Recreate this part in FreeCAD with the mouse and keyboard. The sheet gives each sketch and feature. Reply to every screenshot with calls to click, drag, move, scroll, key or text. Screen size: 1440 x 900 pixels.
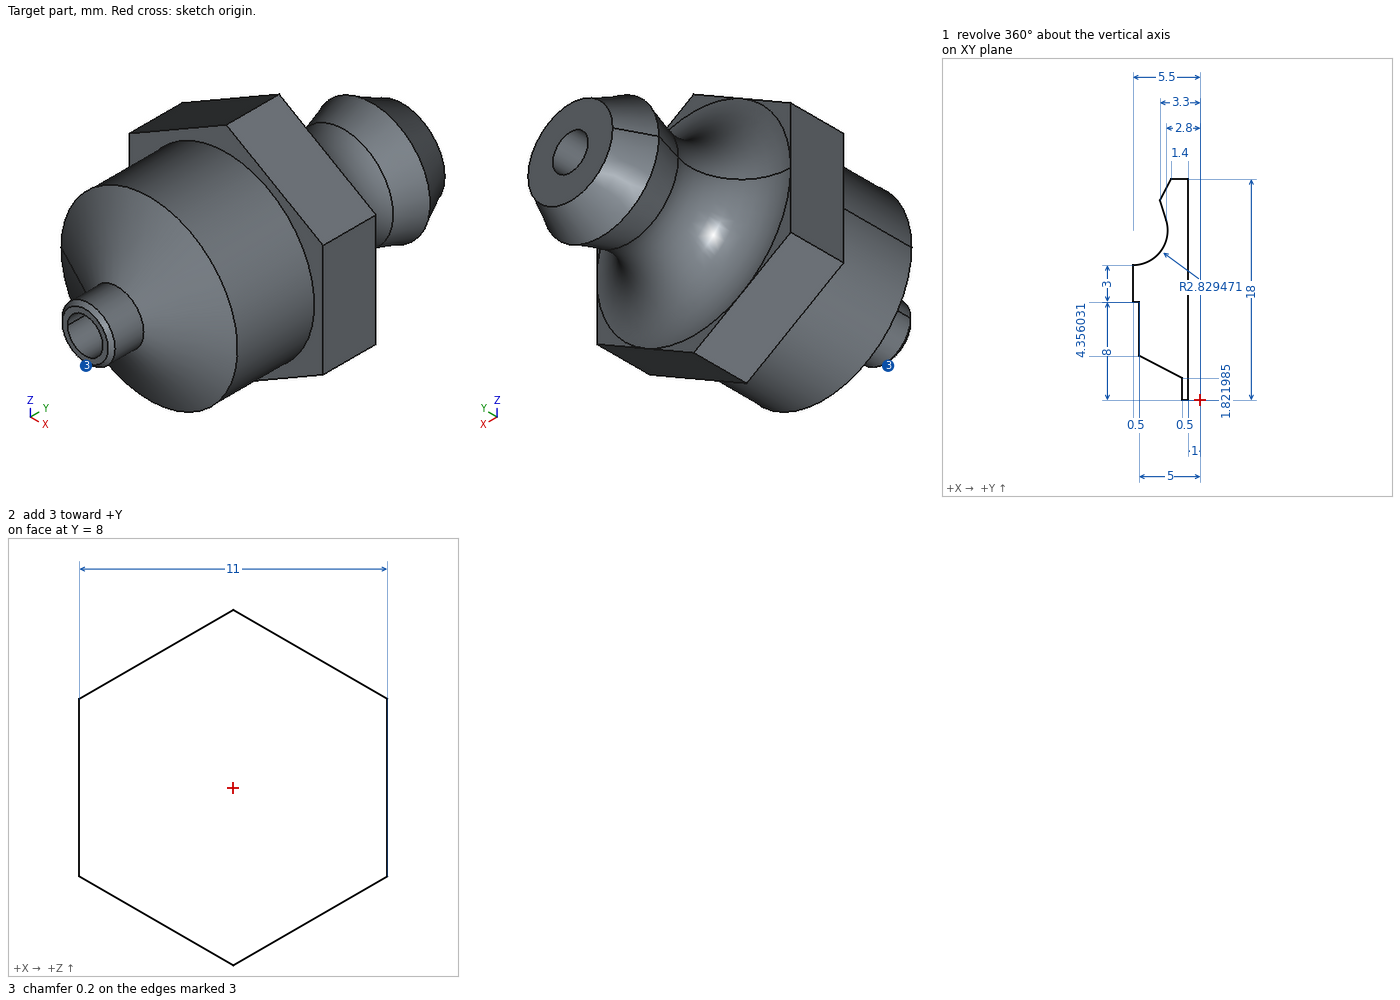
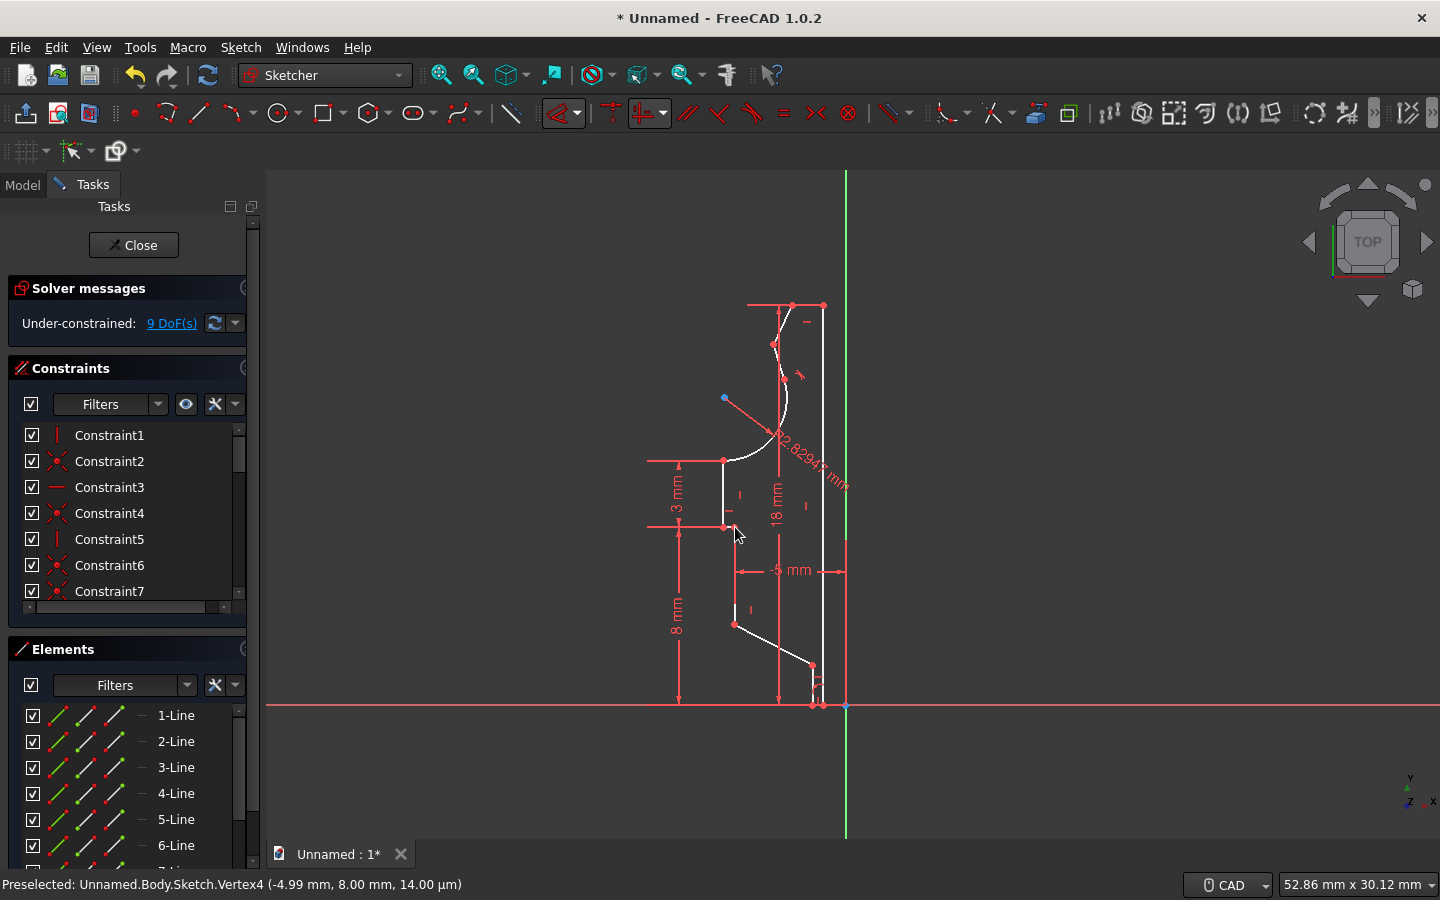
scroll(823, 705, up, 3)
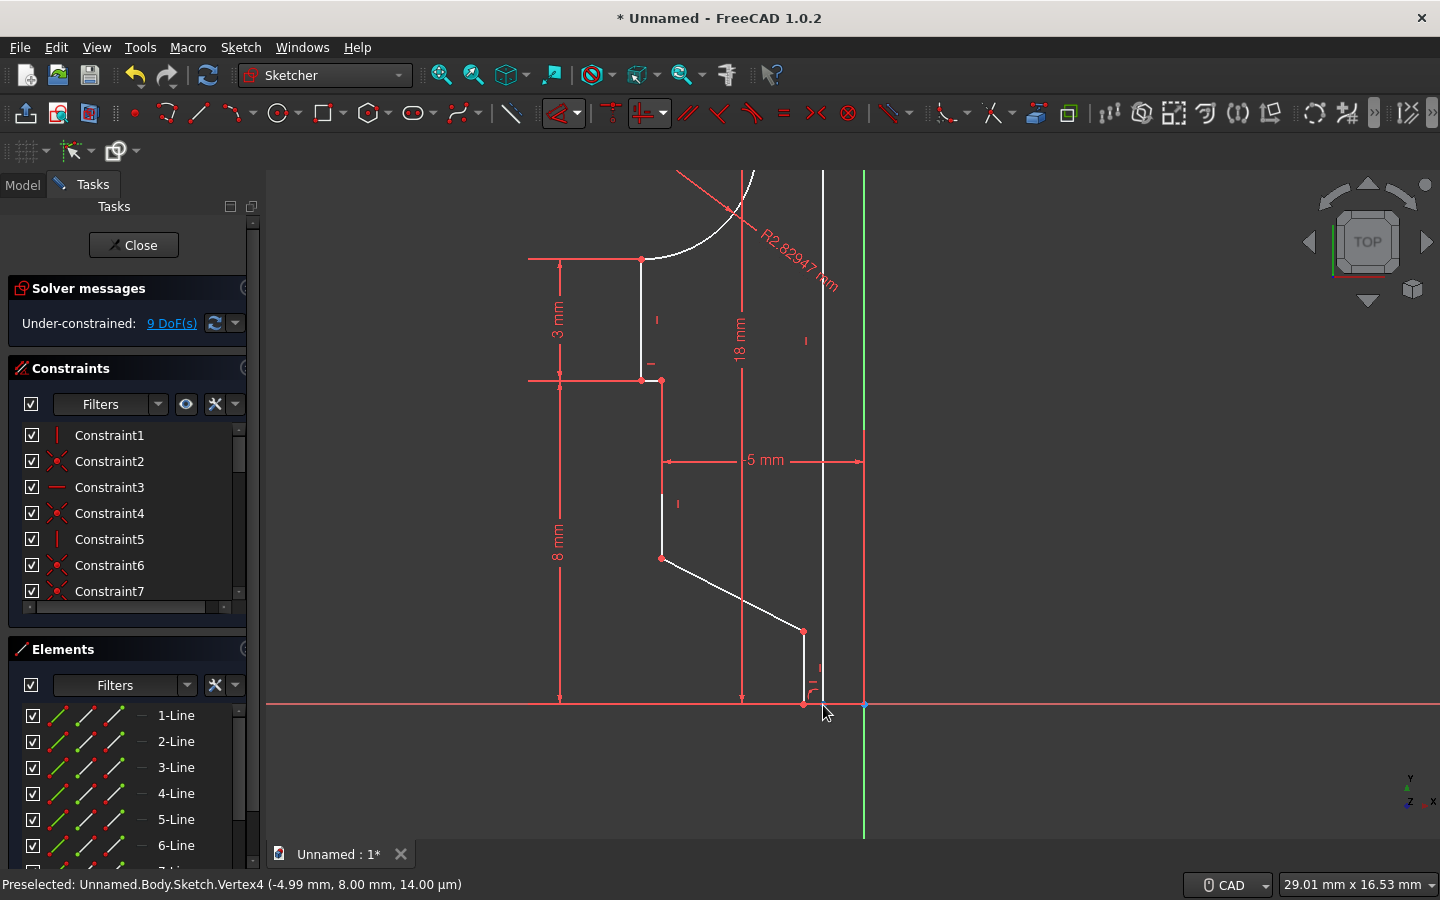
click(823, 704)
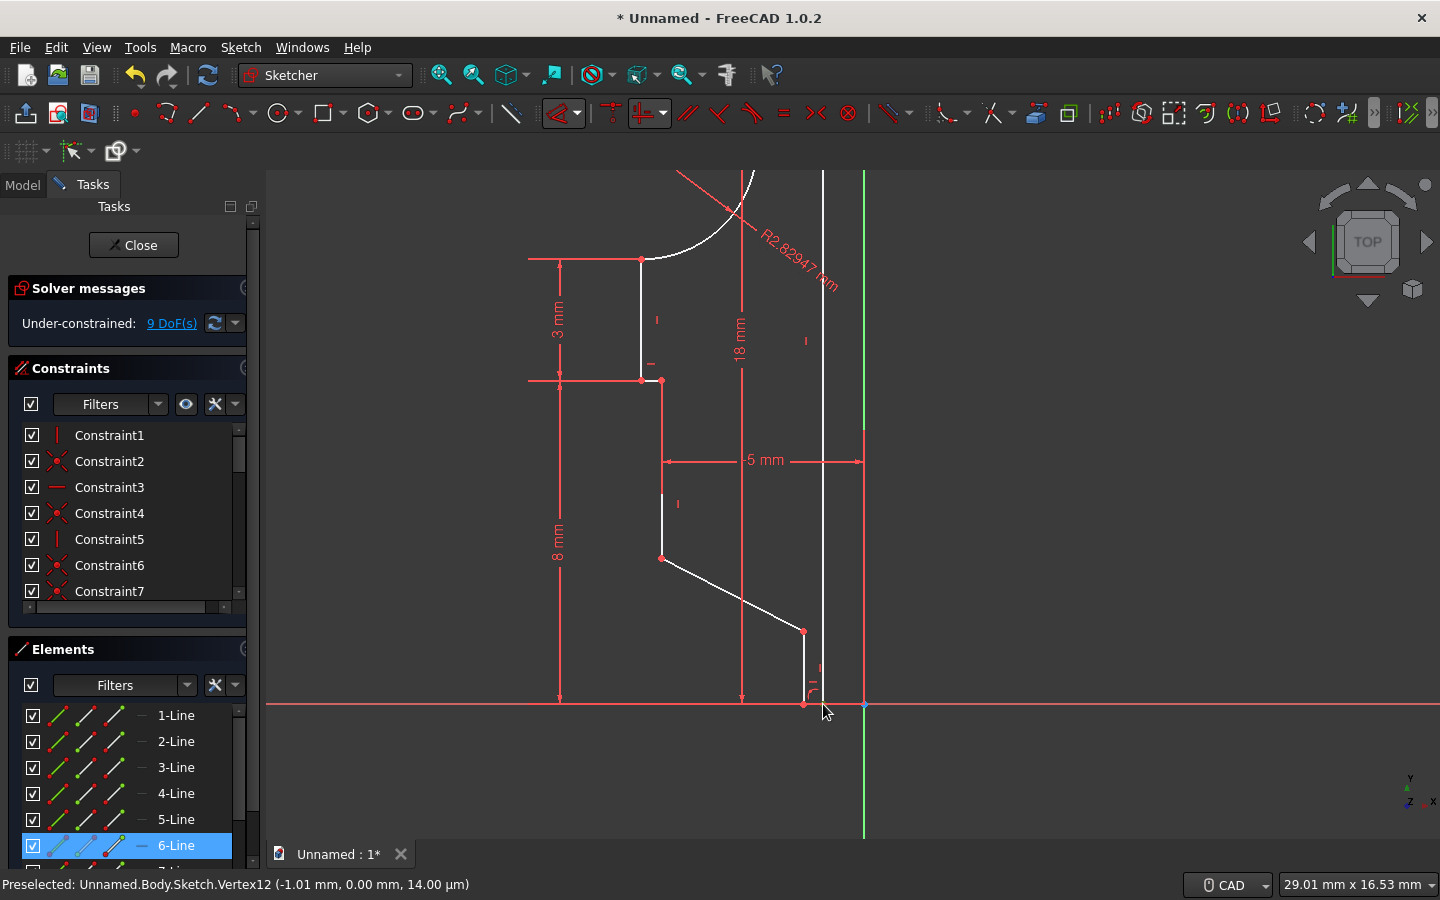
key(l)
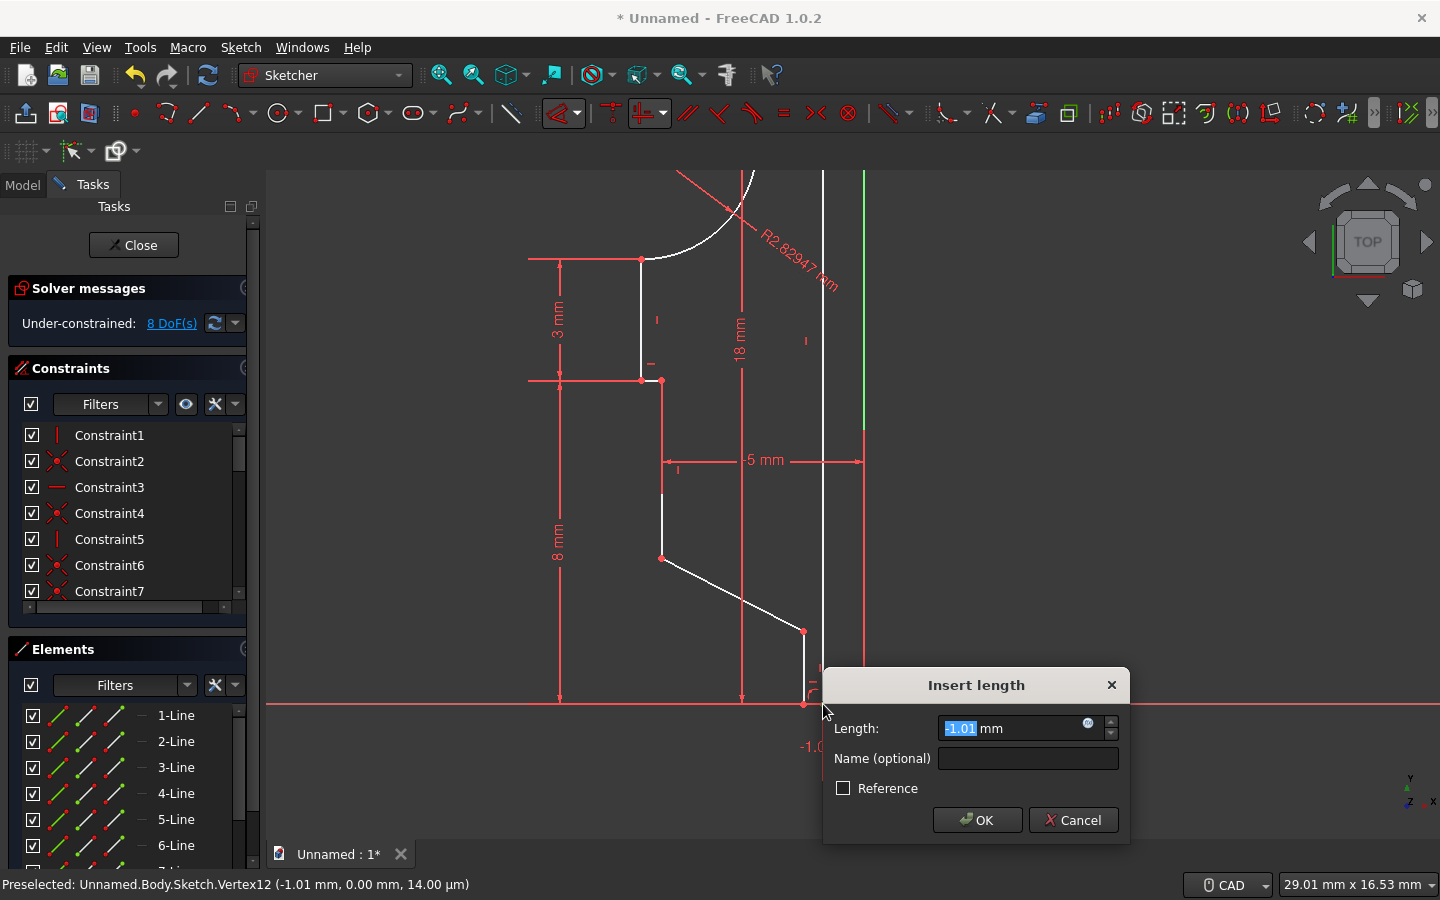
text(-1)
key(Return)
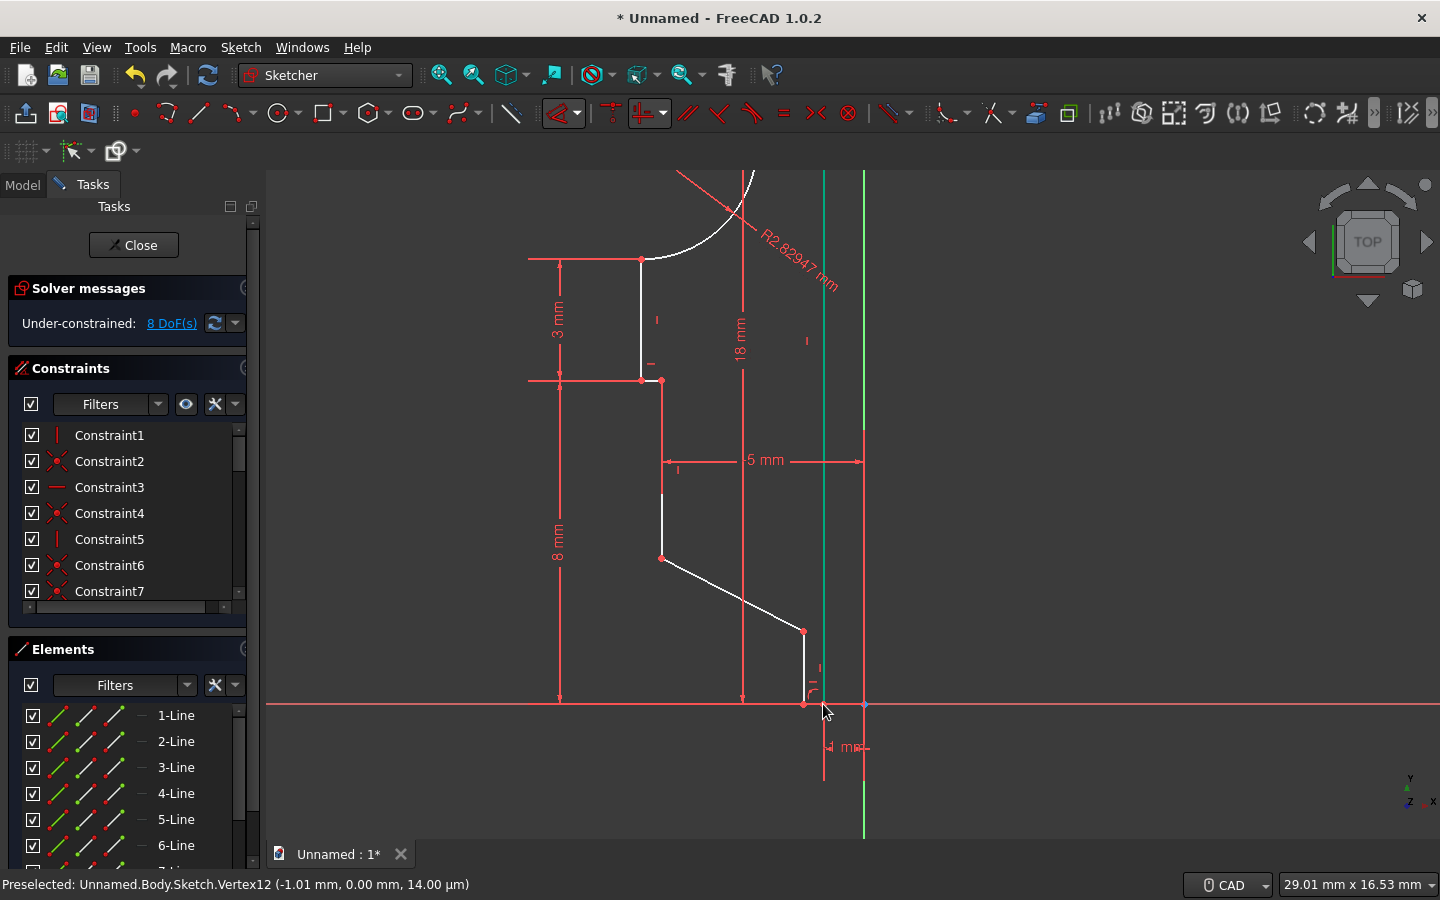
scroll(652, 381, up, 4)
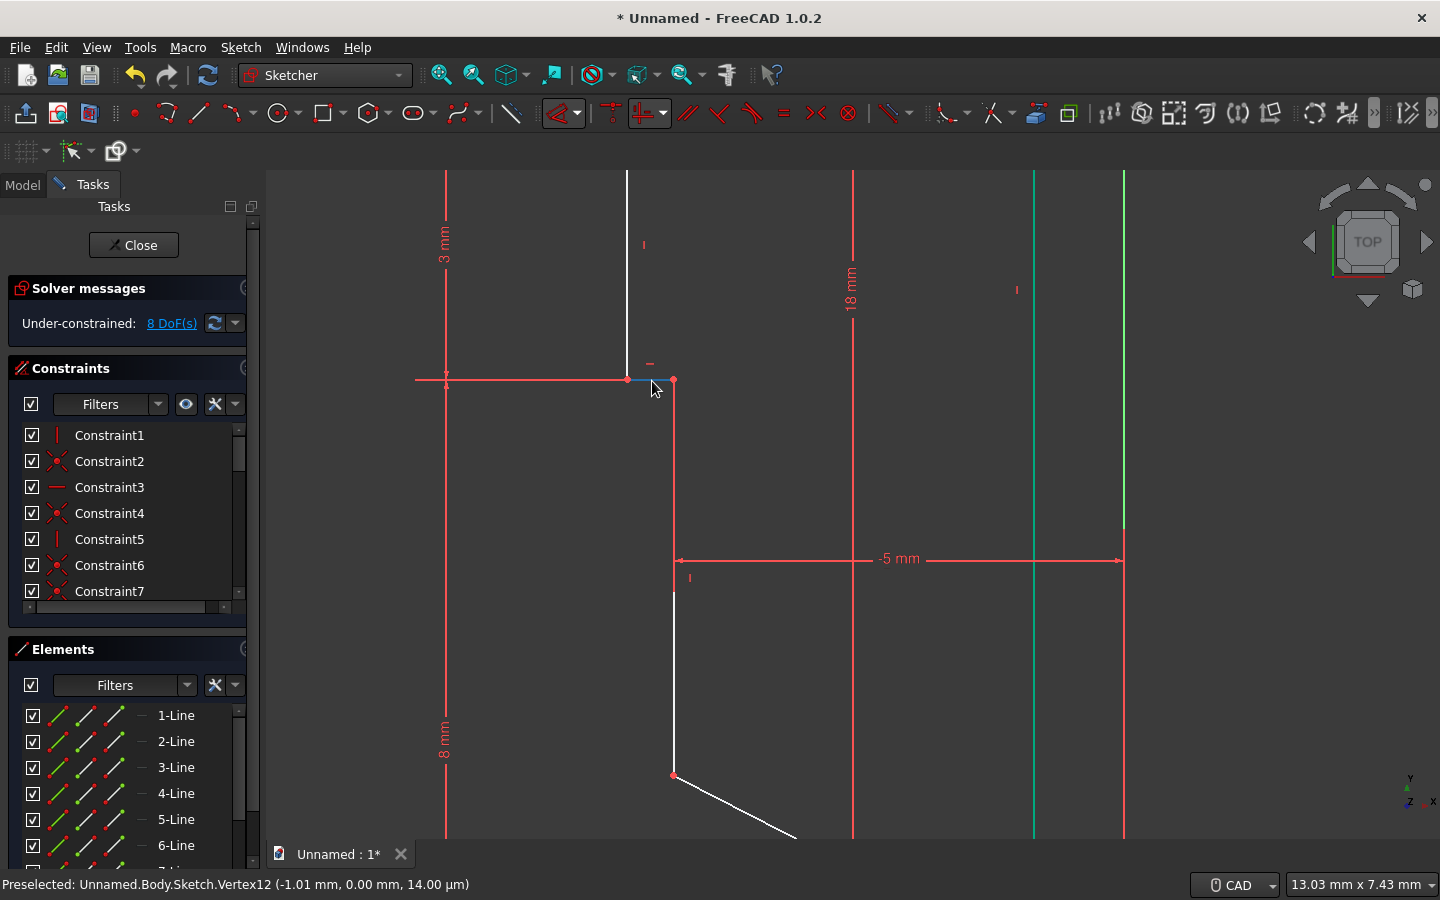
click(651, 380)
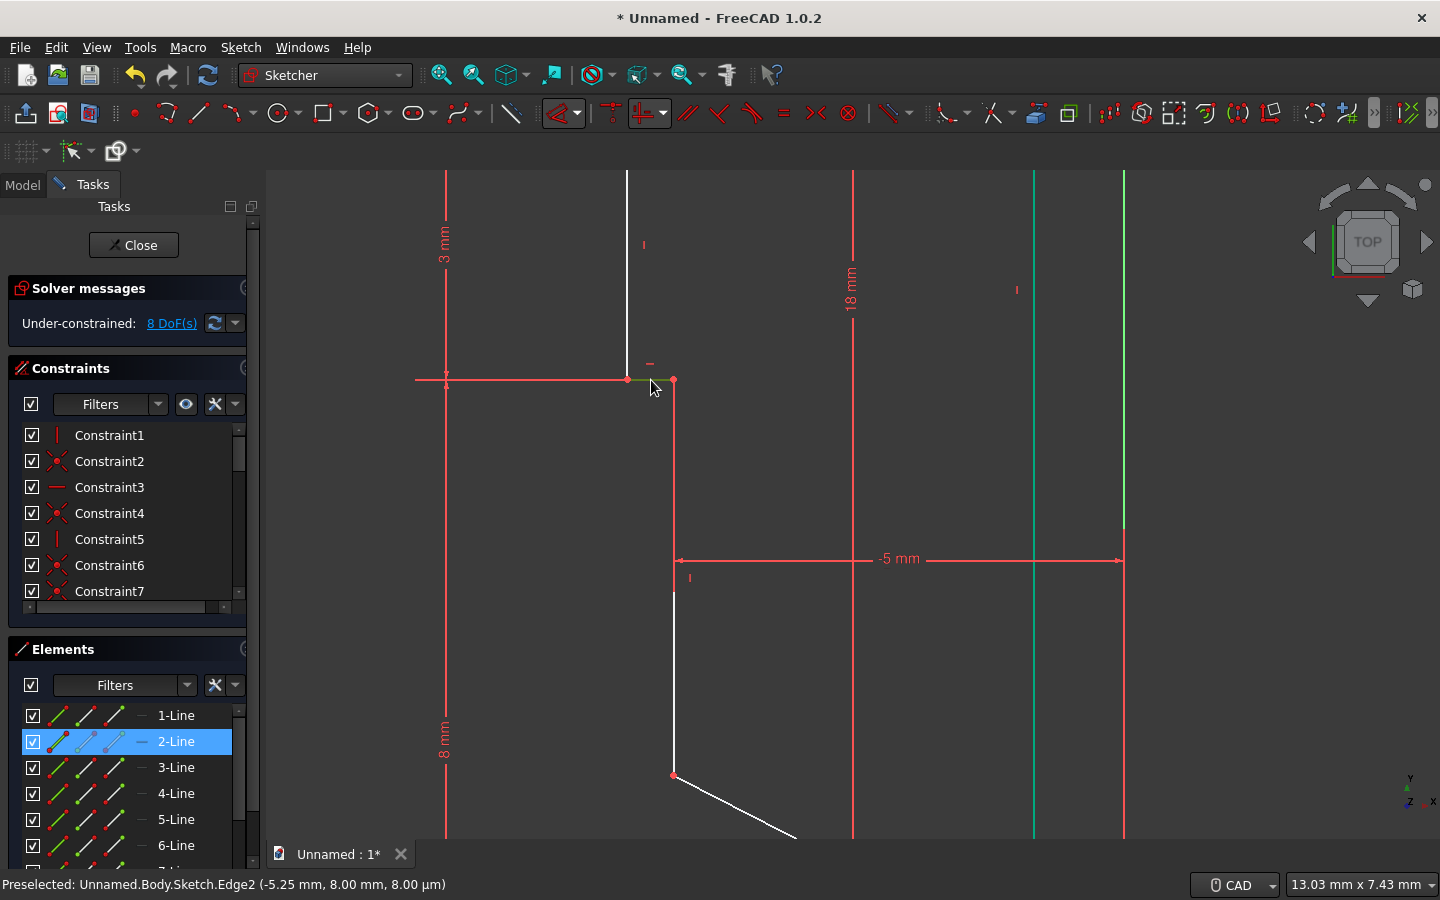
key(l)